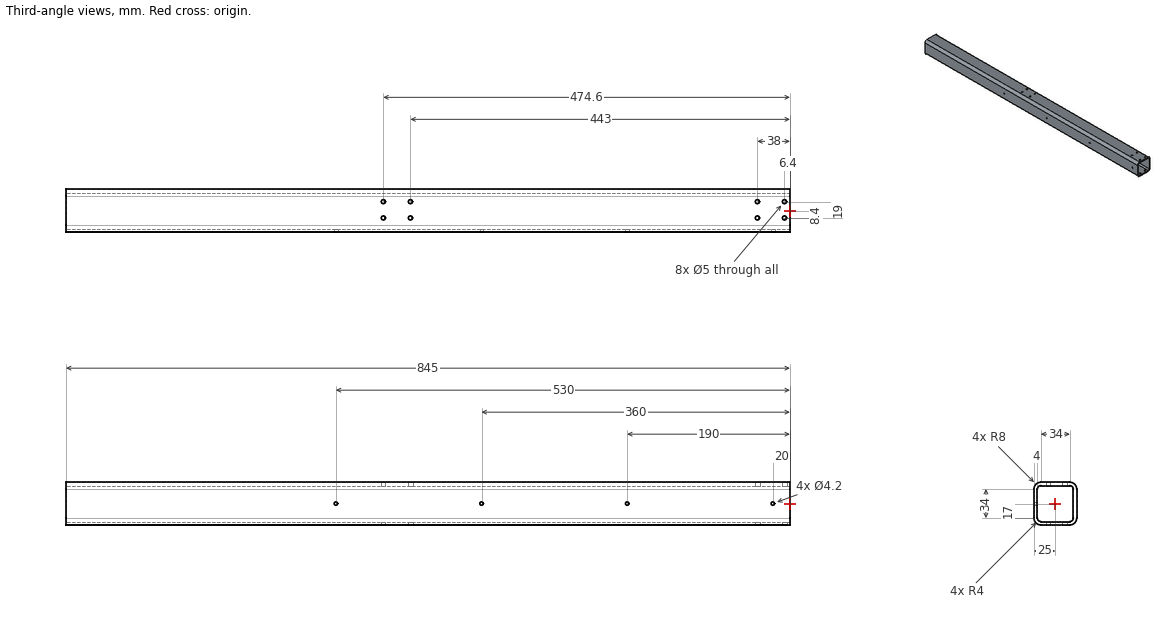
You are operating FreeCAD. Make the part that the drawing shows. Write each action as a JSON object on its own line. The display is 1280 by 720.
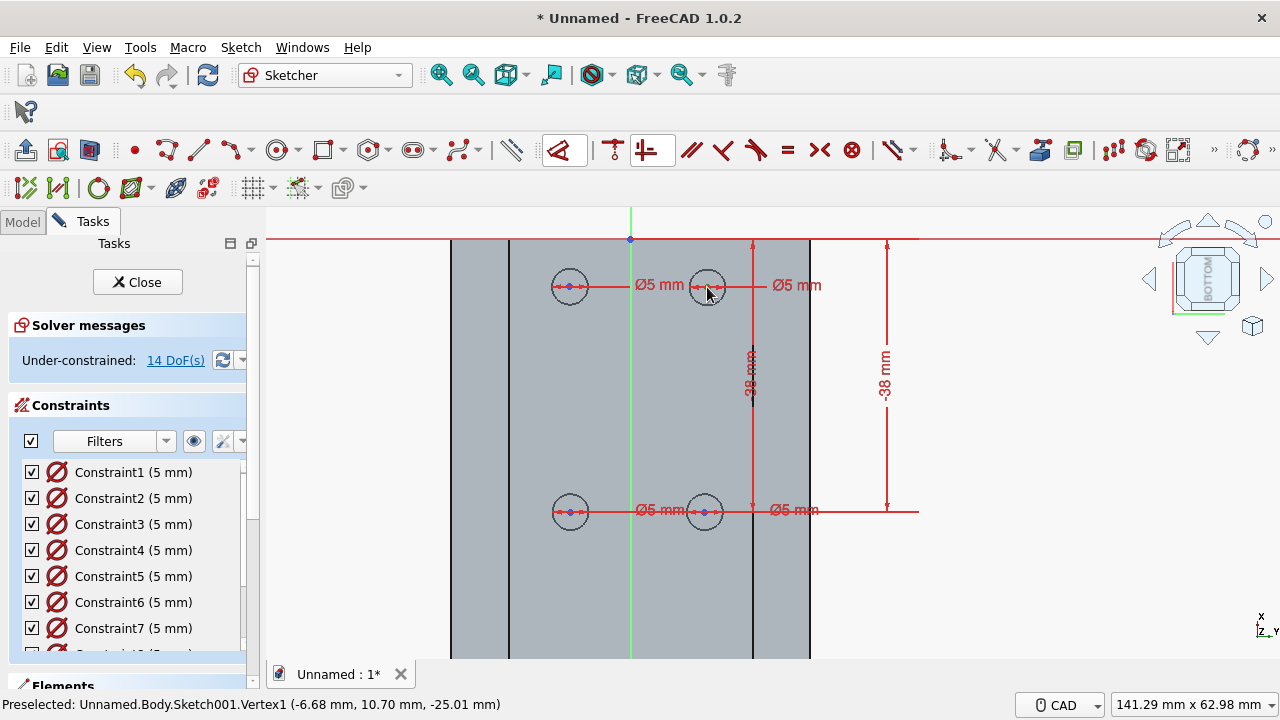
{"action": "left_click", "coordinate": [582, 150]}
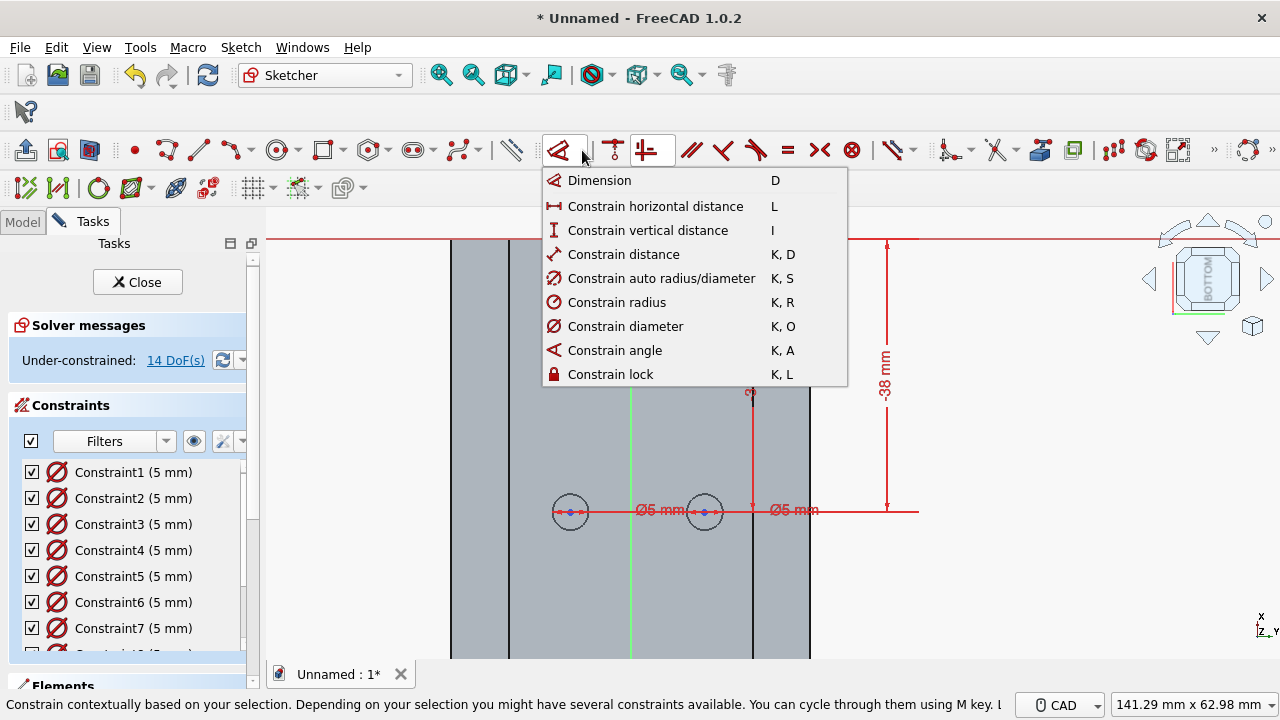
{"action": "left_click", "coordinate": [695, 230]}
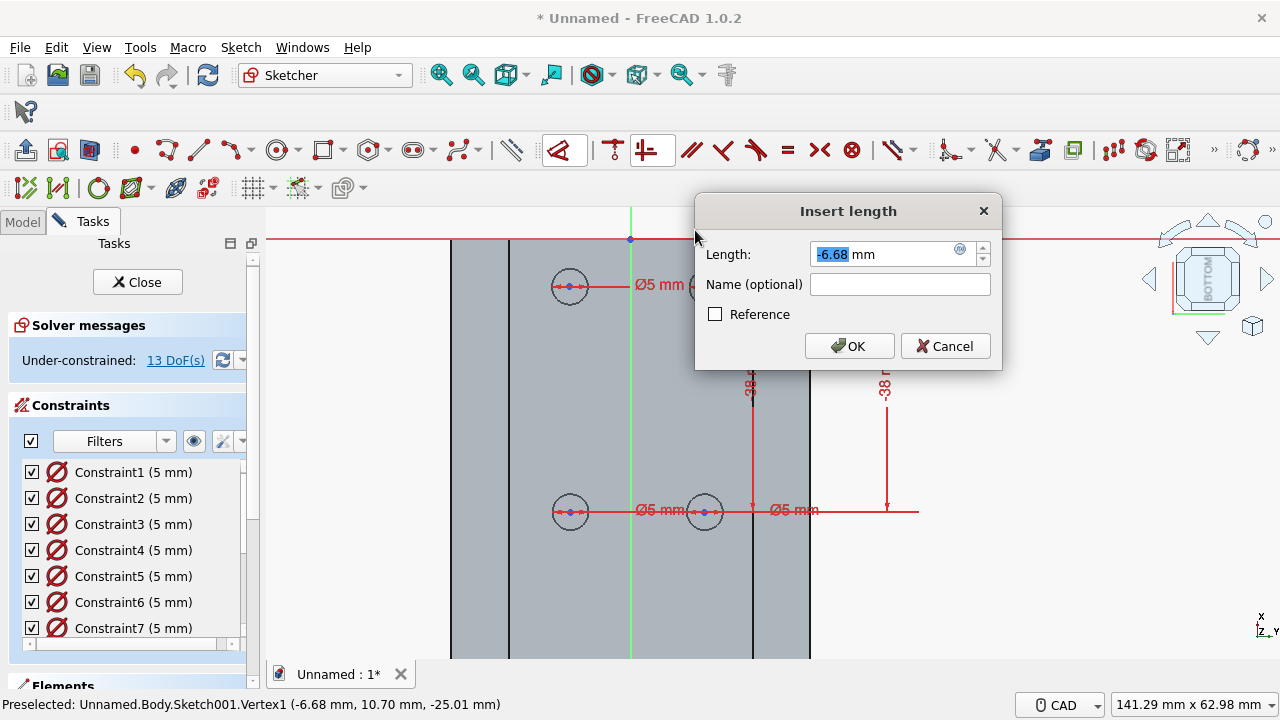
{"action": "type", "text": "-6.4"}
{"action": "key", "text": "Return"}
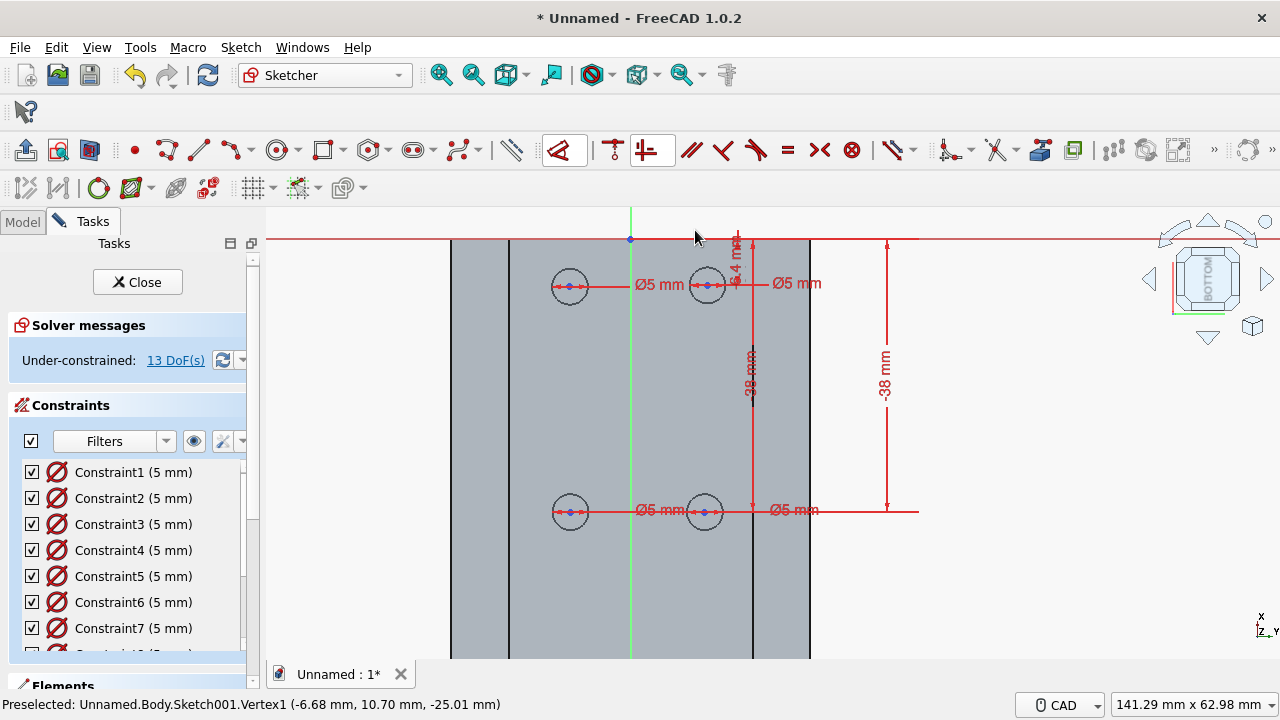
{"action": "left_click", "coordinate": [570, 287]}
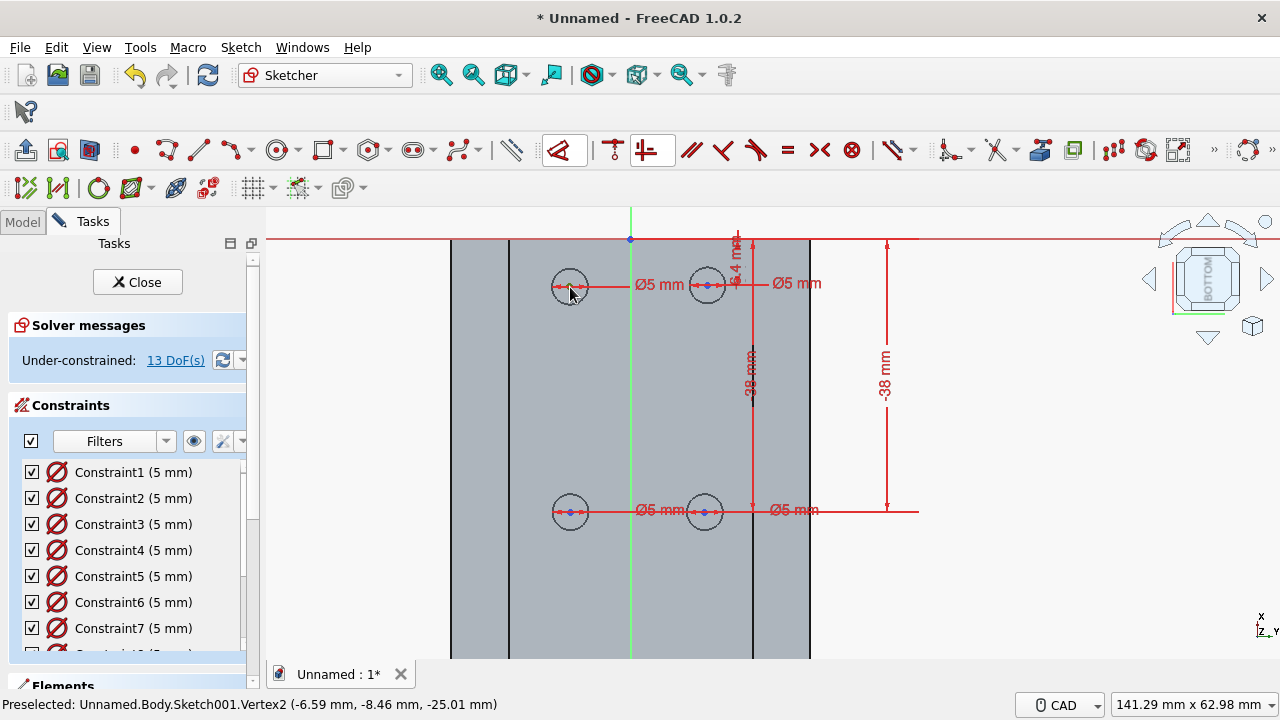
{"action": "left_click", "coordinate": [582, 150]}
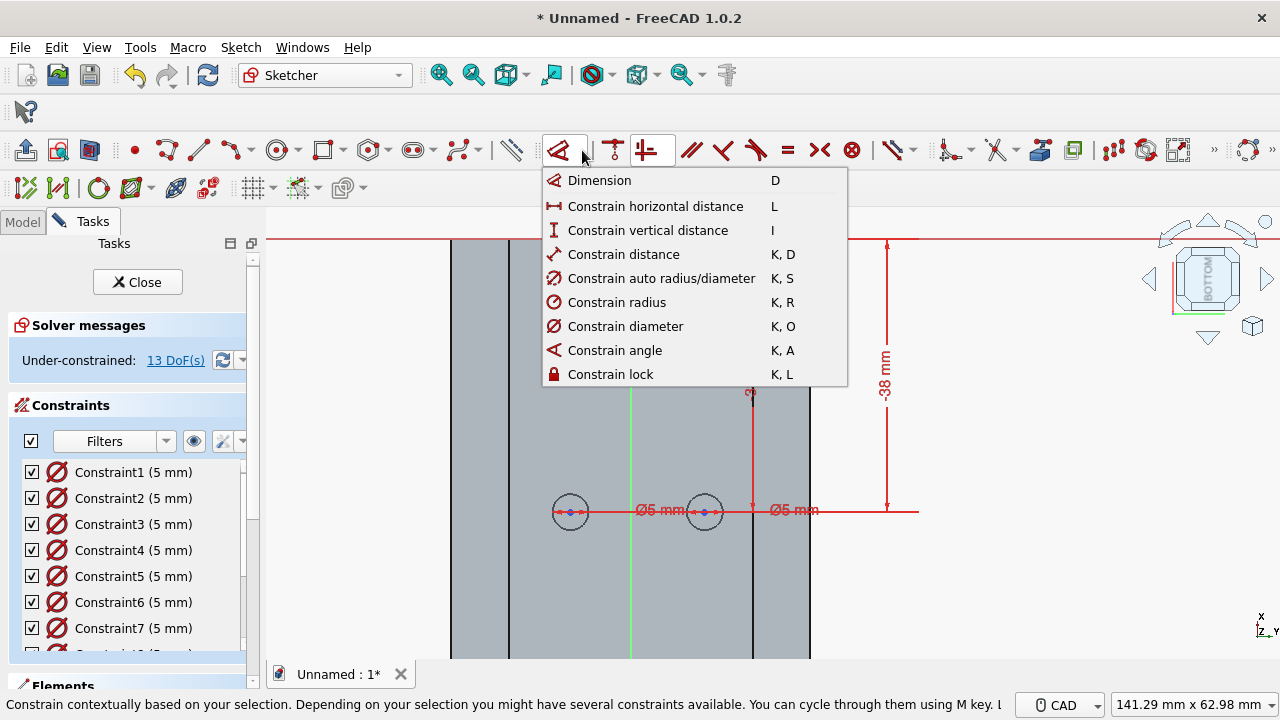
{"action": "left_click", "coordinate": [695, 206]}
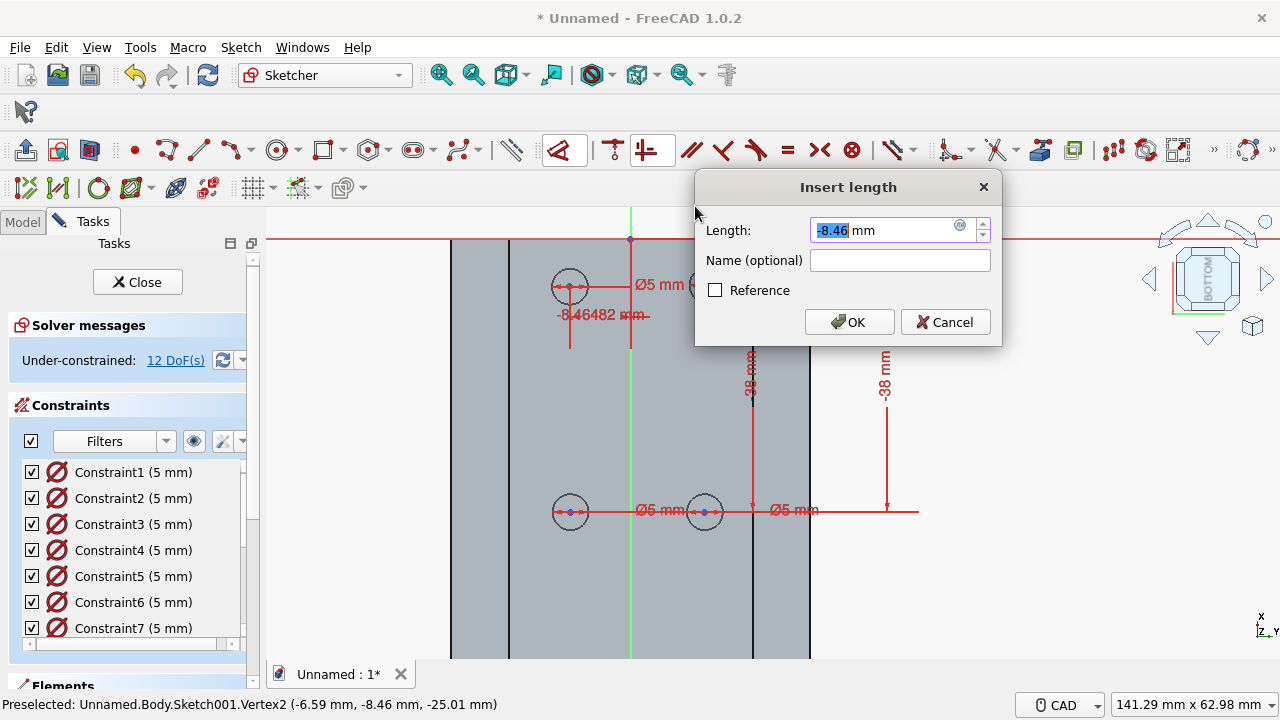
{"action": "type", "text": "-8.4"}
{"action": "key", "text": "Return"}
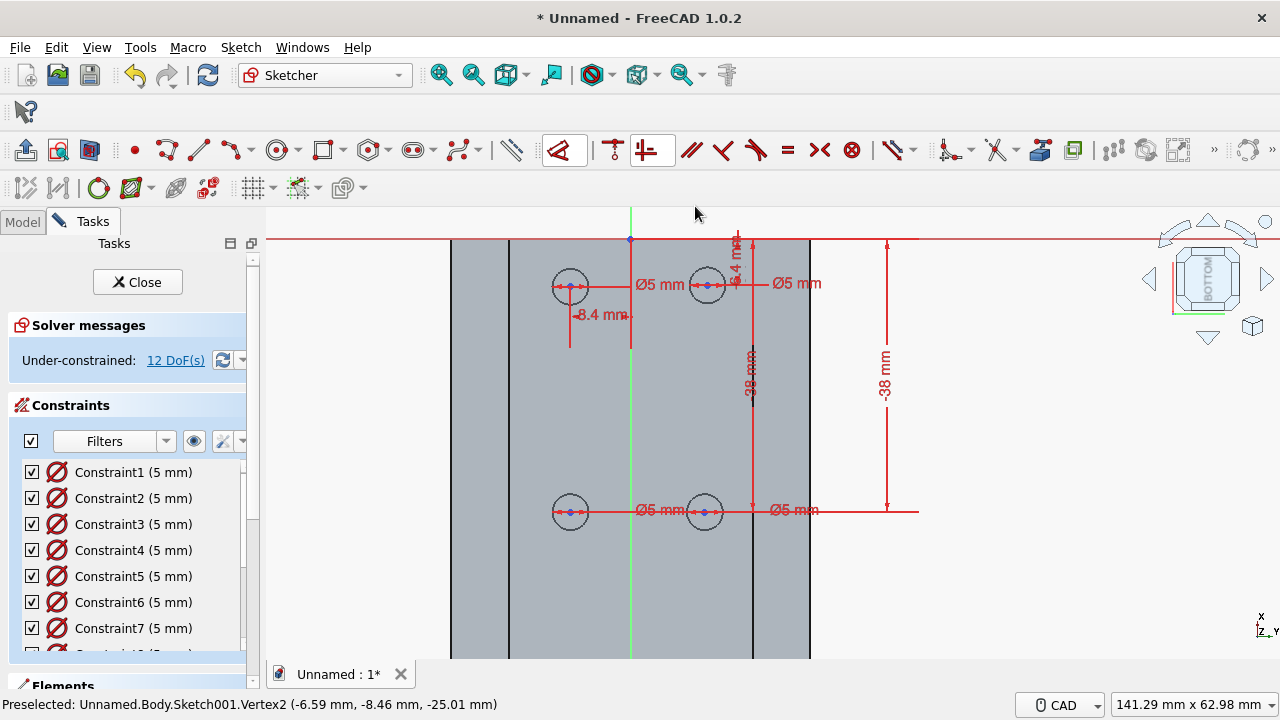
{"action": "left_click", "coordinate": [570, 287]}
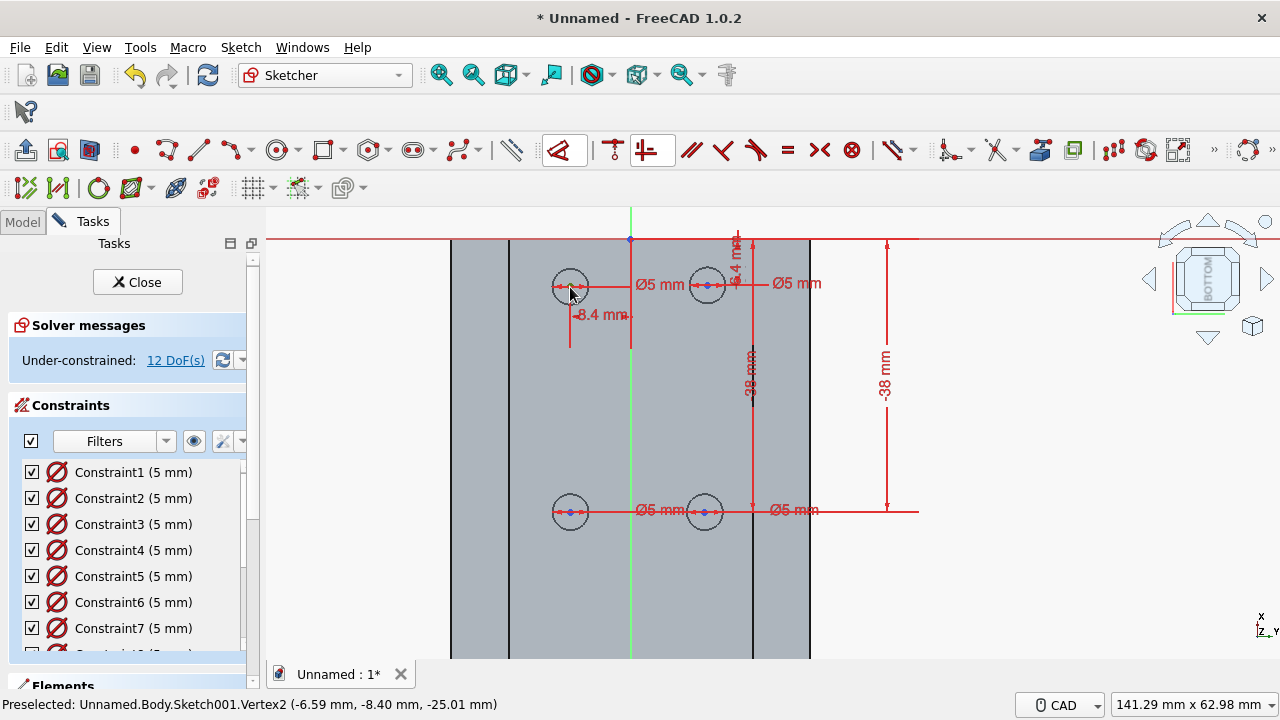
{"action": "key", "text": "i"}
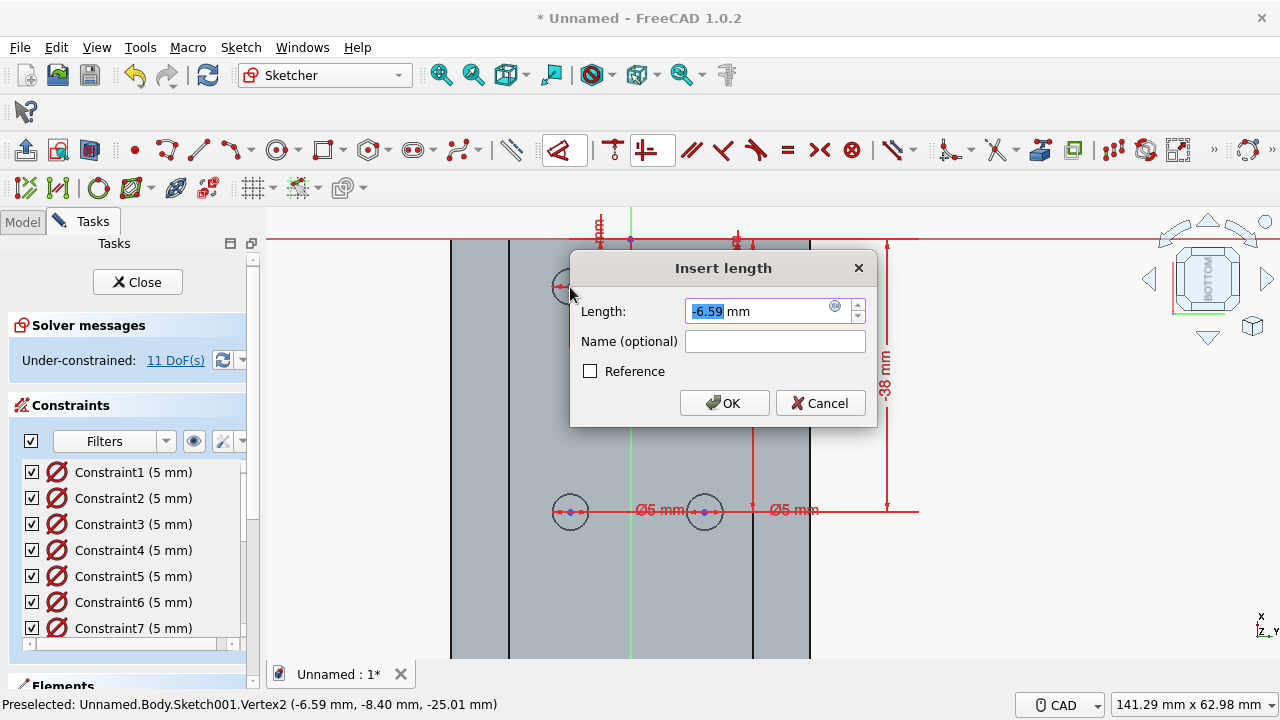
{"action": "type", "text": "-6.4"}
{"action": "key", "text": "Return"}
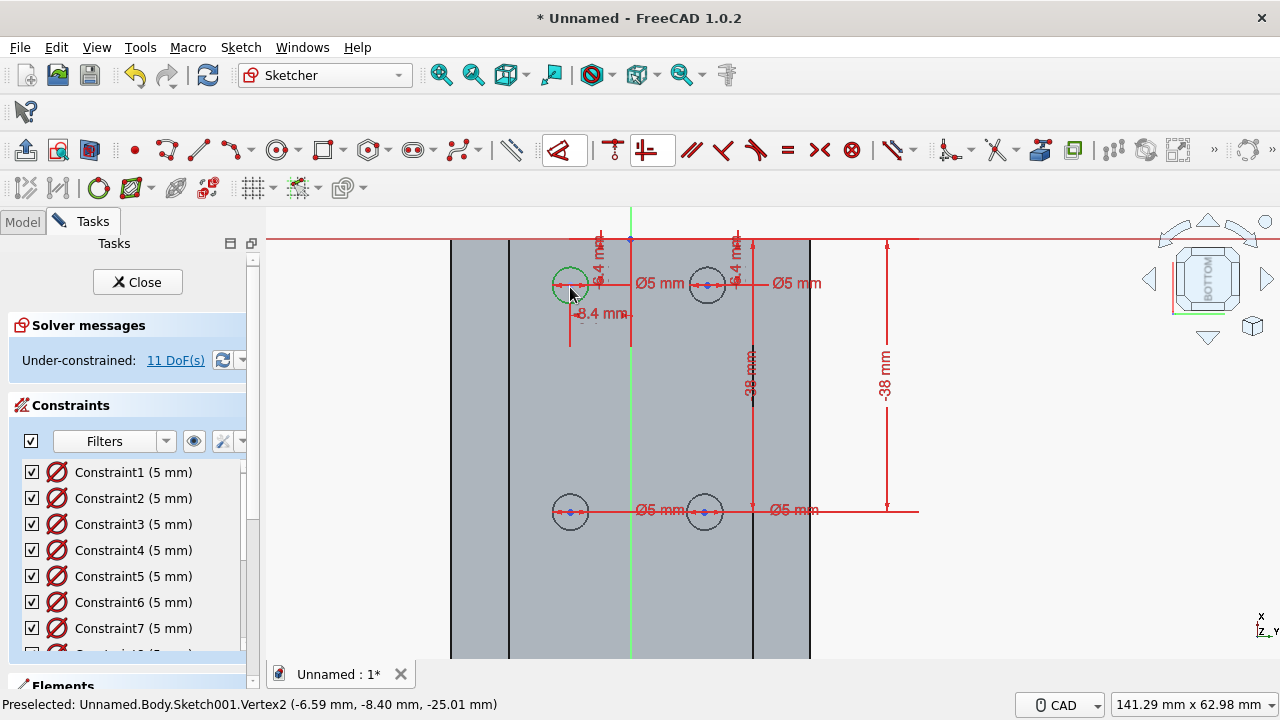
{"action": "left_click", "coordinate": [571, 512]}